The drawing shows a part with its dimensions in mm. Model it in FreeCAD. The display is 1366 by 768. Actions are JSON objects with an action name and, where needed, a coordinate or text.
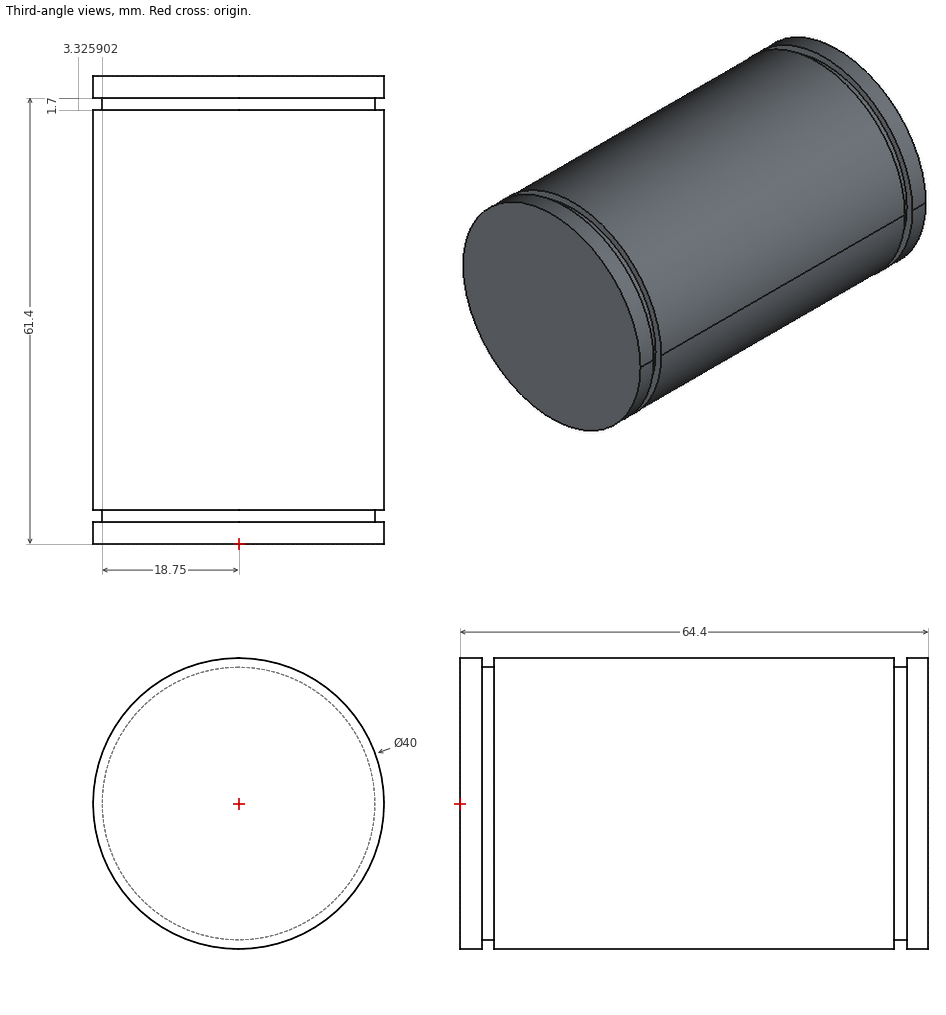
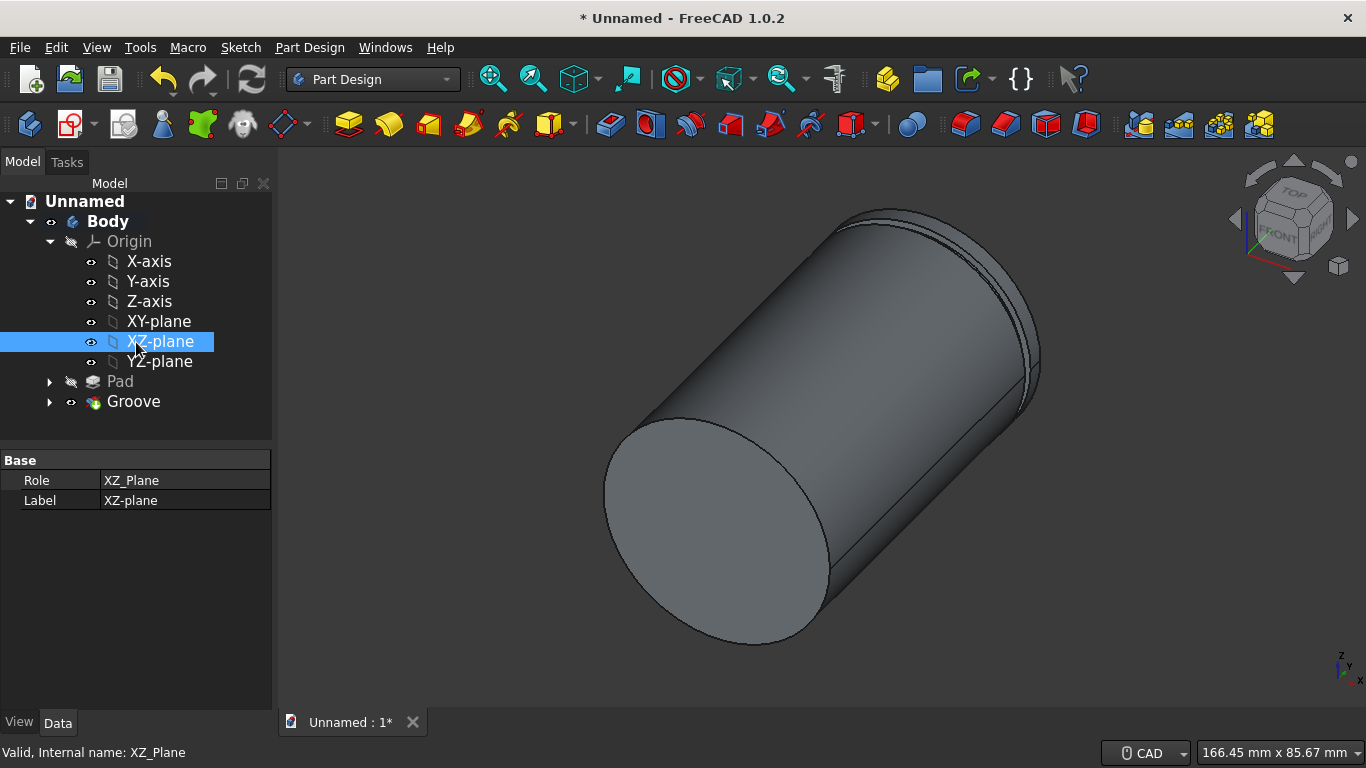
{"action": "left_click", "coordinate": [284, 124]}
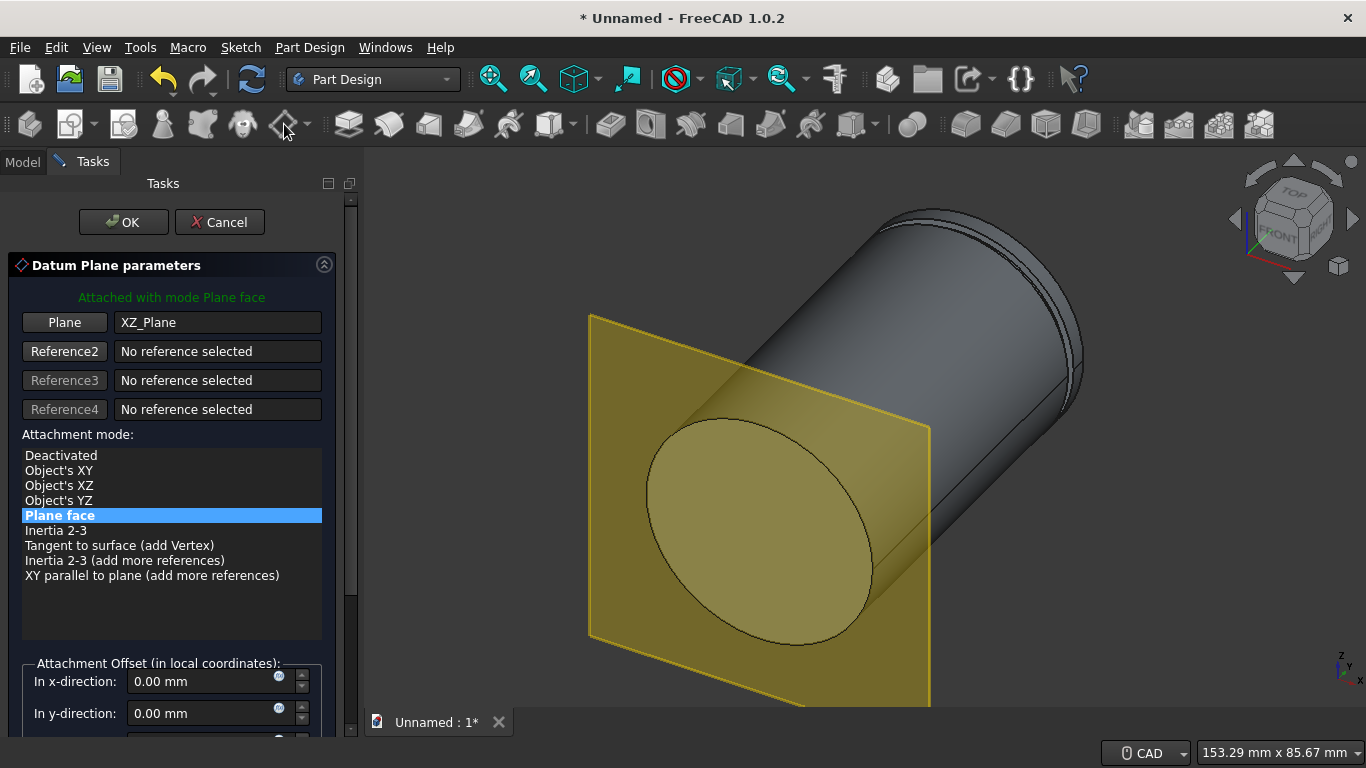
{"action": "scroll", "coordinate": [351, 464], "scroll_direction": "down", "scroll_amount": 2}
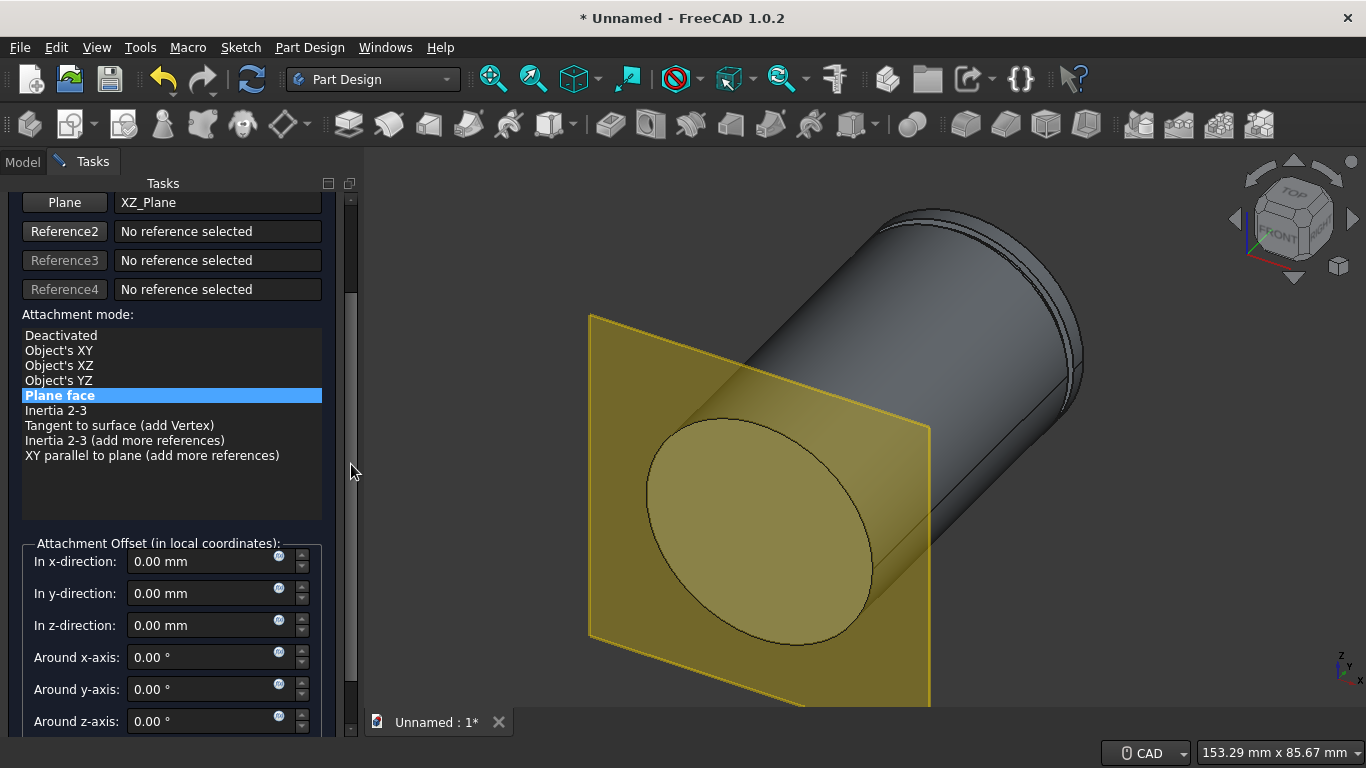
{"action": "triple_click", "coordinate": [210, 625]}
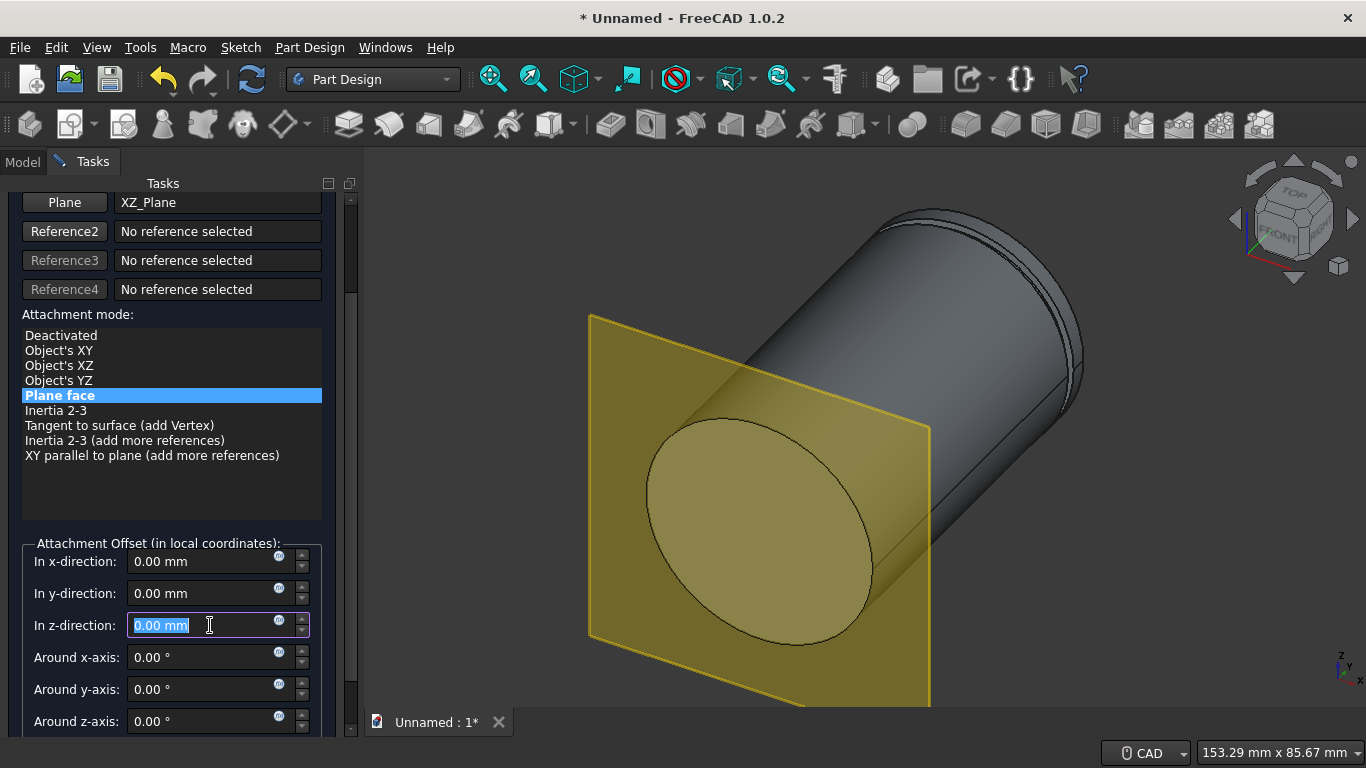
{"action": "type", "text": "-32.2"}
{"action": "key", "text": "Tab"}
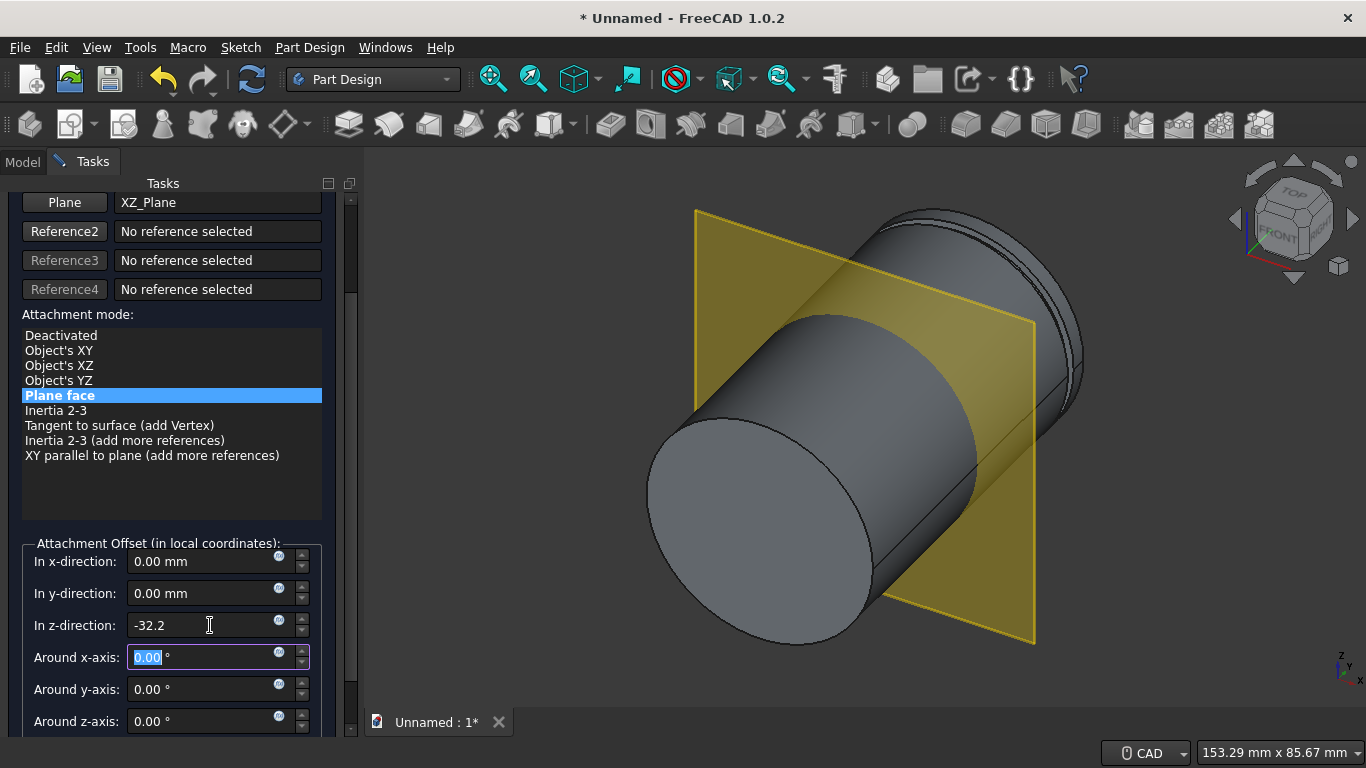
{"action": "scroll", "coordinate": [351, 464], "scroll_direction": "up", "scroll_amount": 3}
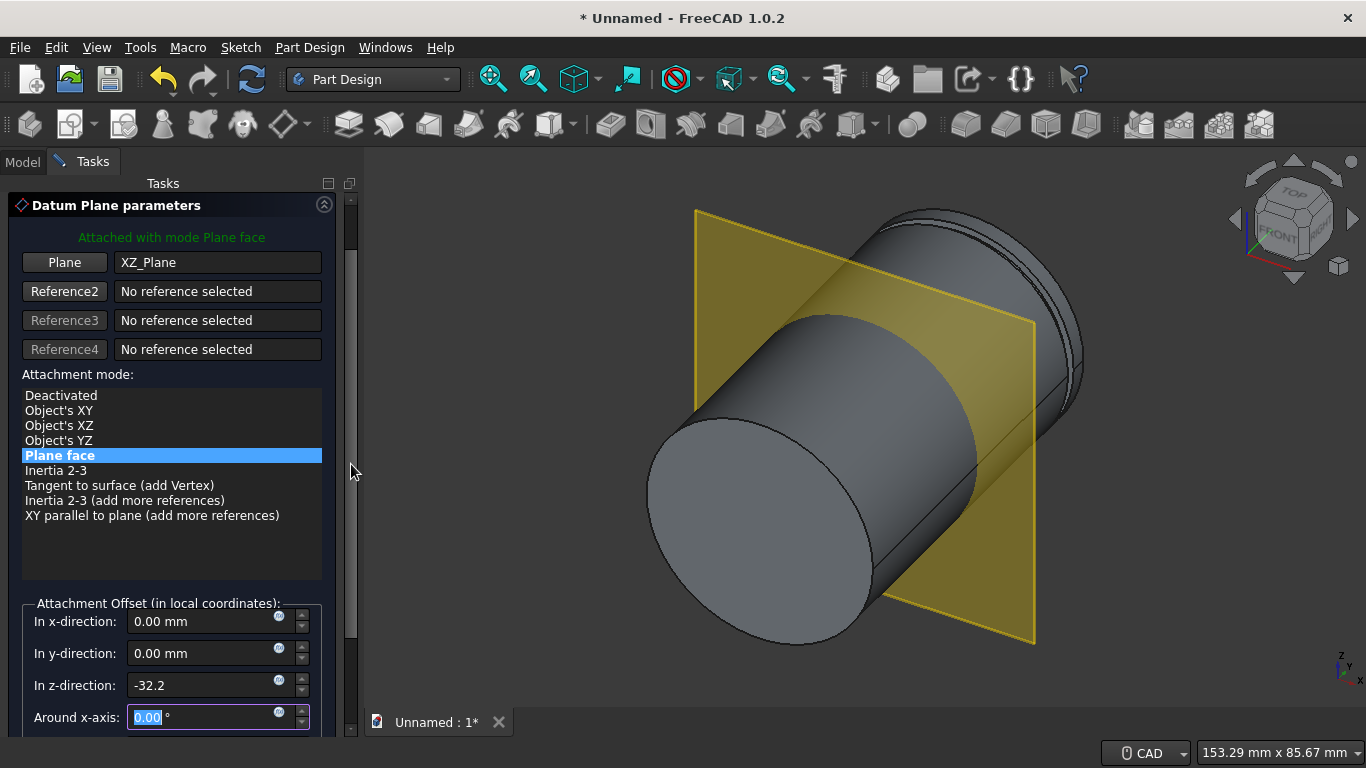
{"action": "left_click", "coordinate": [124, 222]}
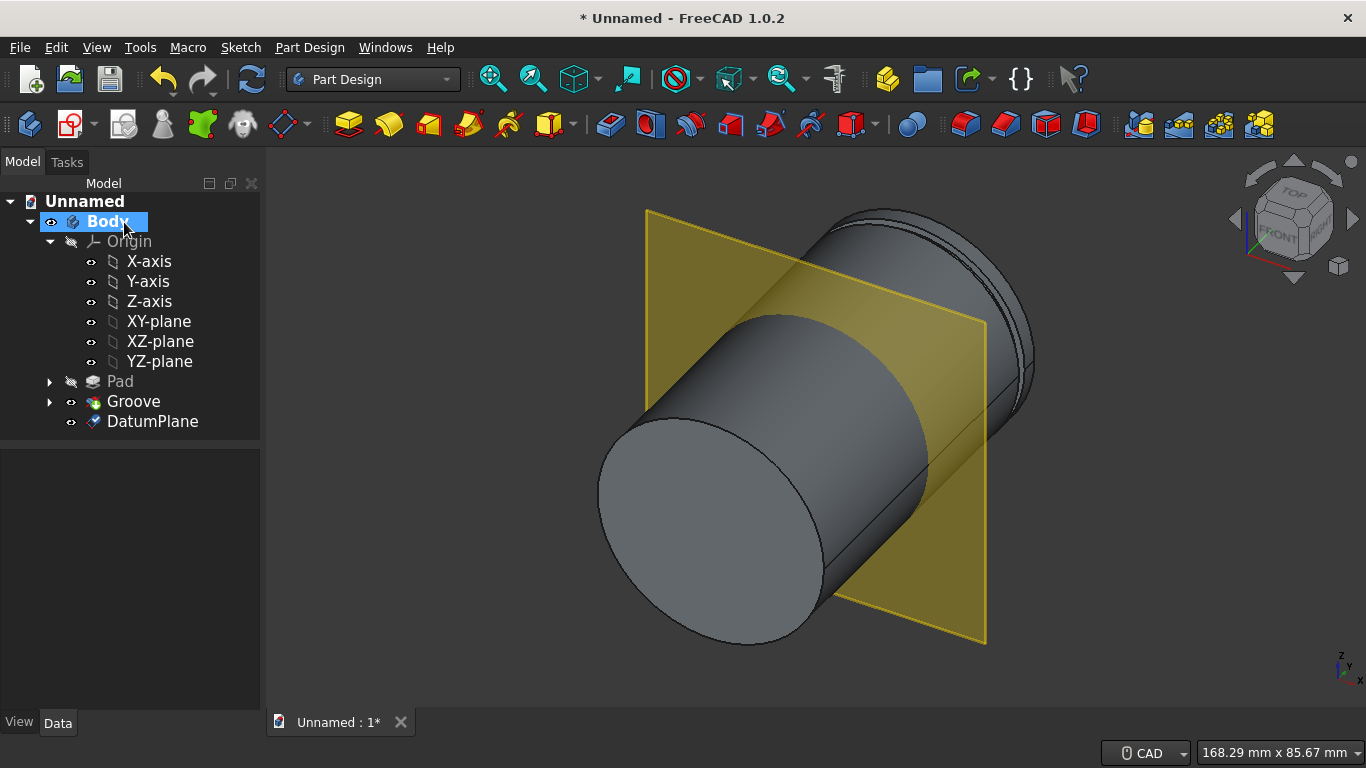
{"action": "left_click", "coordinate": [116, 402]}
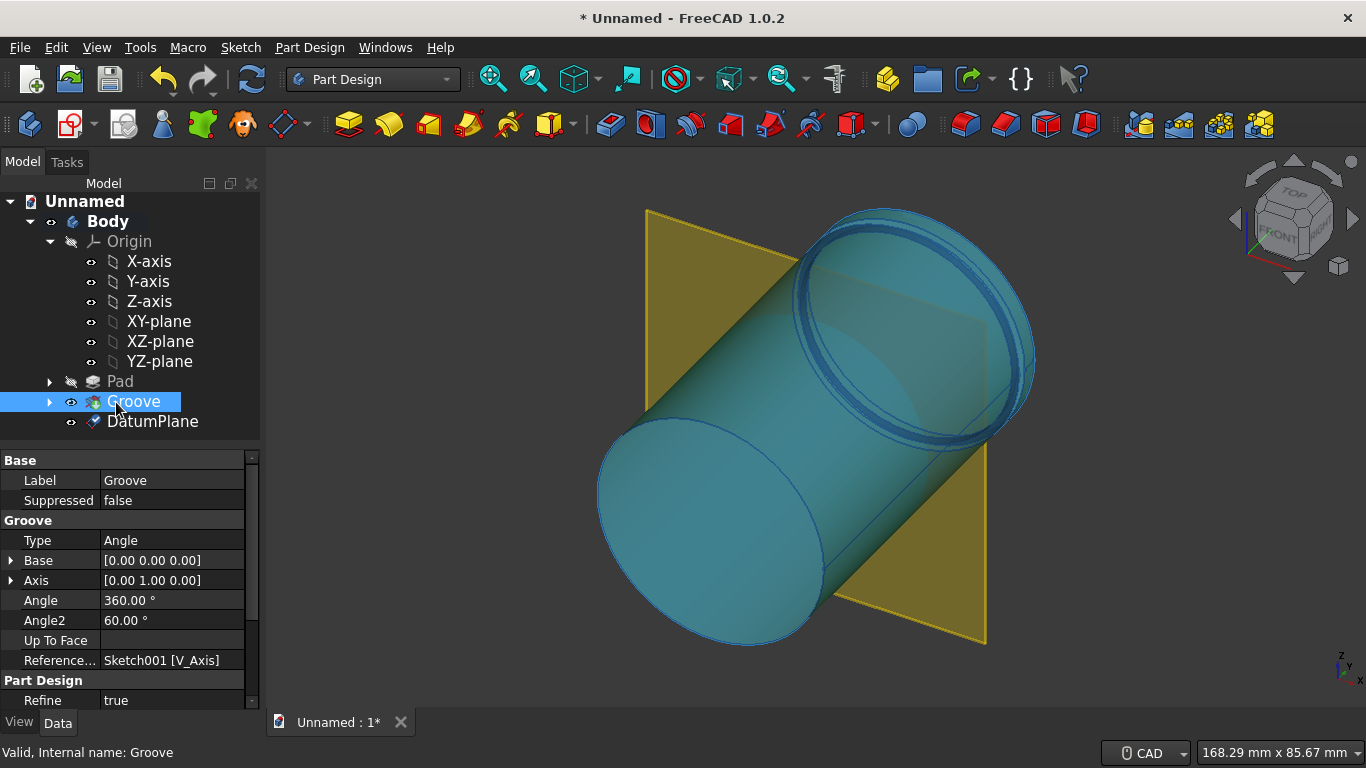
{"action": "left_click", "coordinate": [1140, 124]}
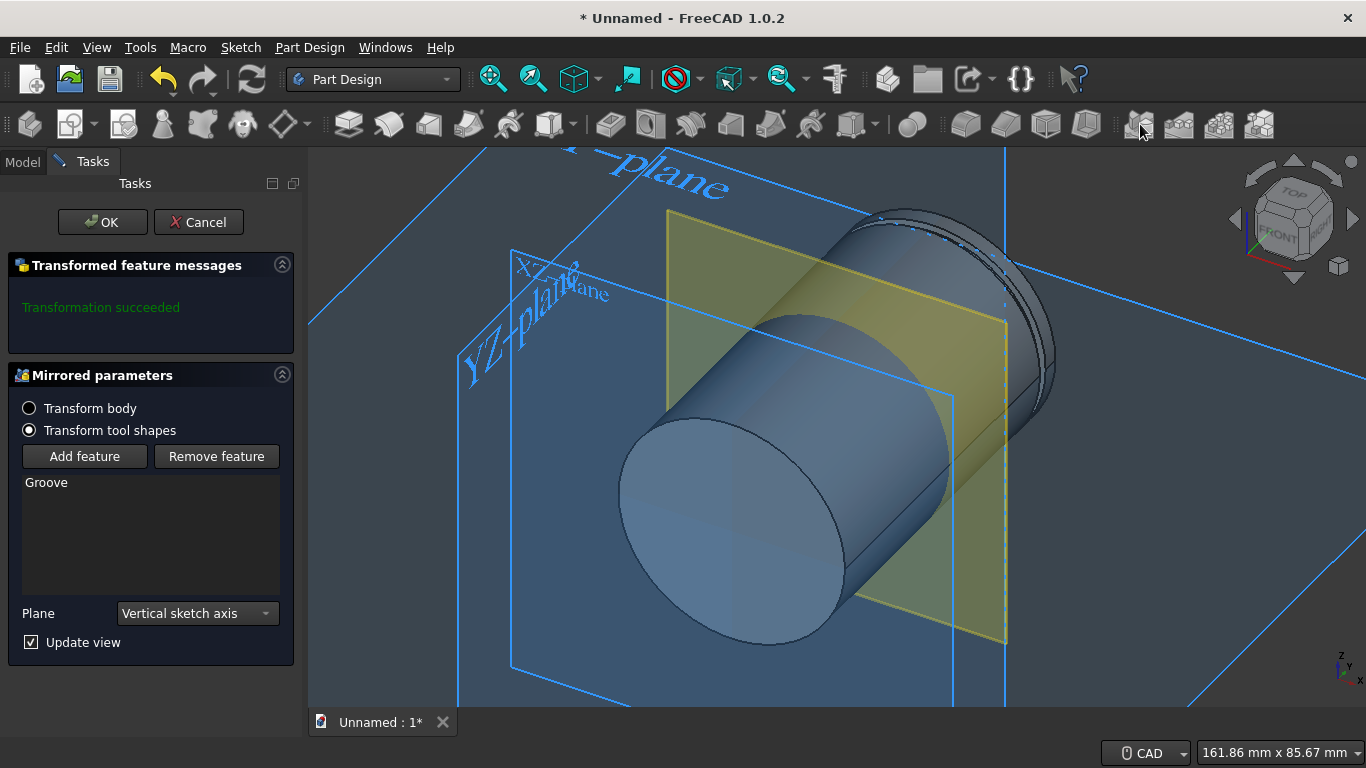
{"action": "left_click", "coordinate": [198, 614]}